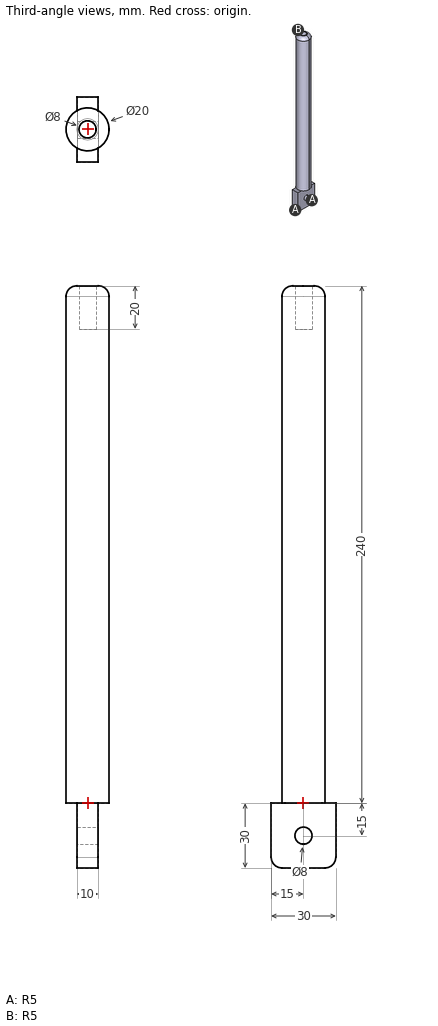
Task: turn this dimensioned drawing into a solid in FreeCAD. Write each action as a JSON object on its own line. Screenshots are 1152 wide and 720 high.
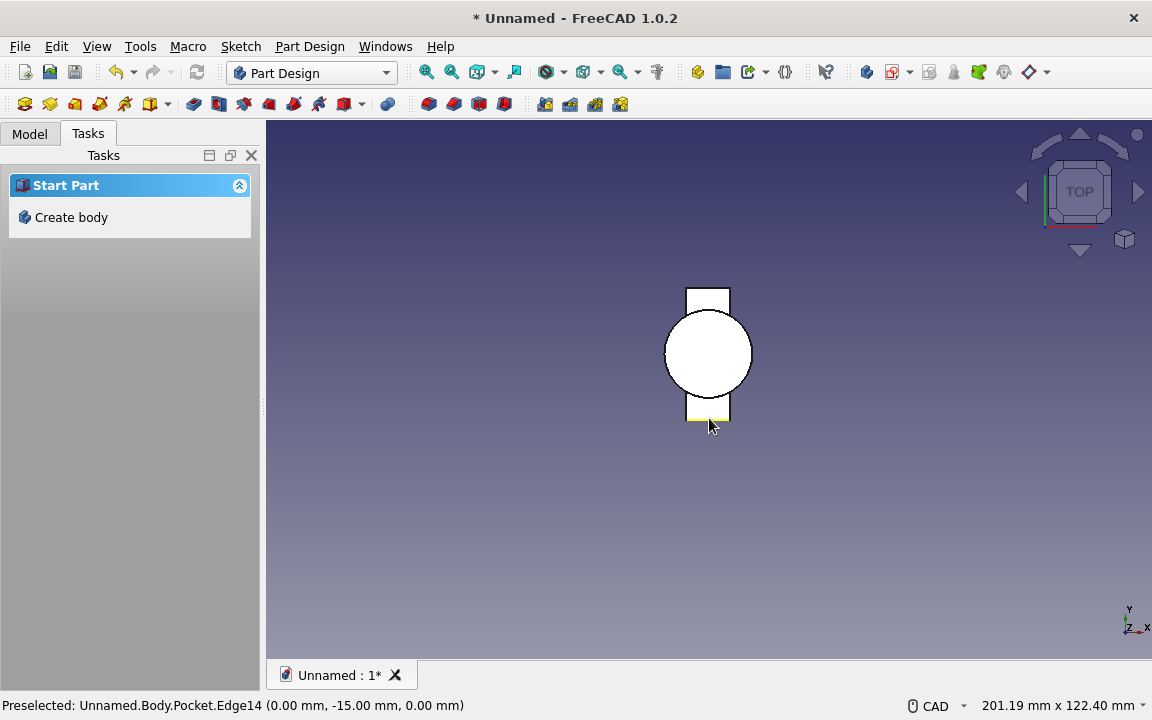
{"action": "key", "text": "v f"}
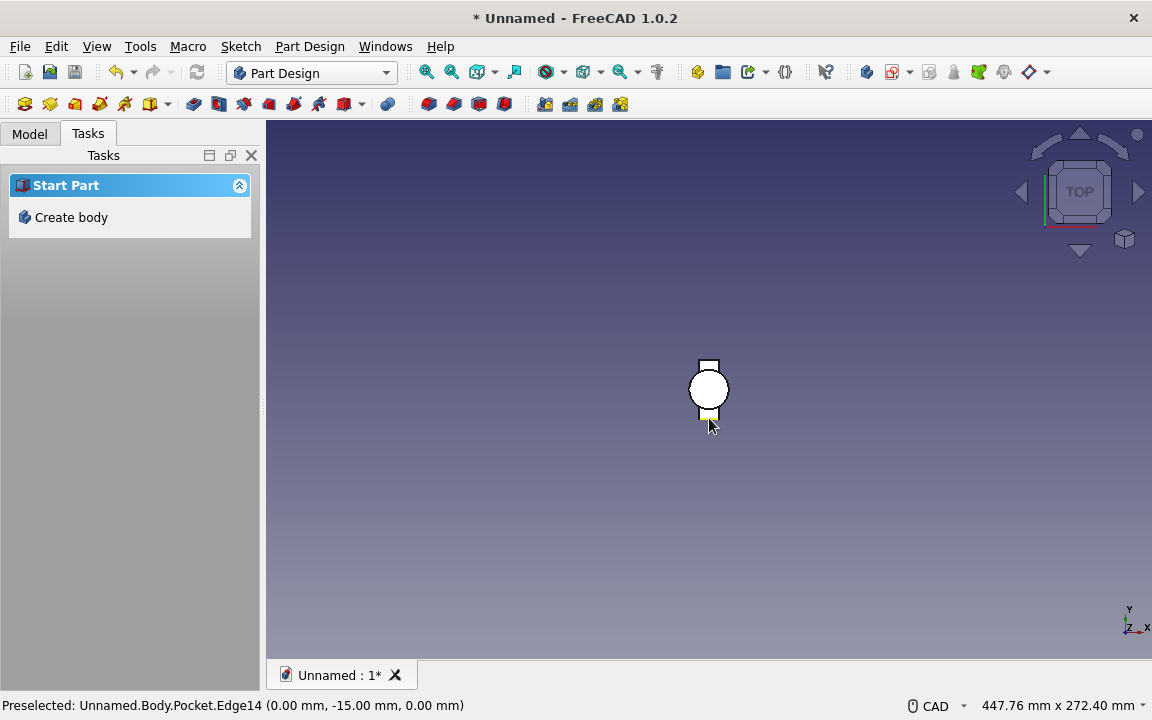
{"action": "key", "text": "1"}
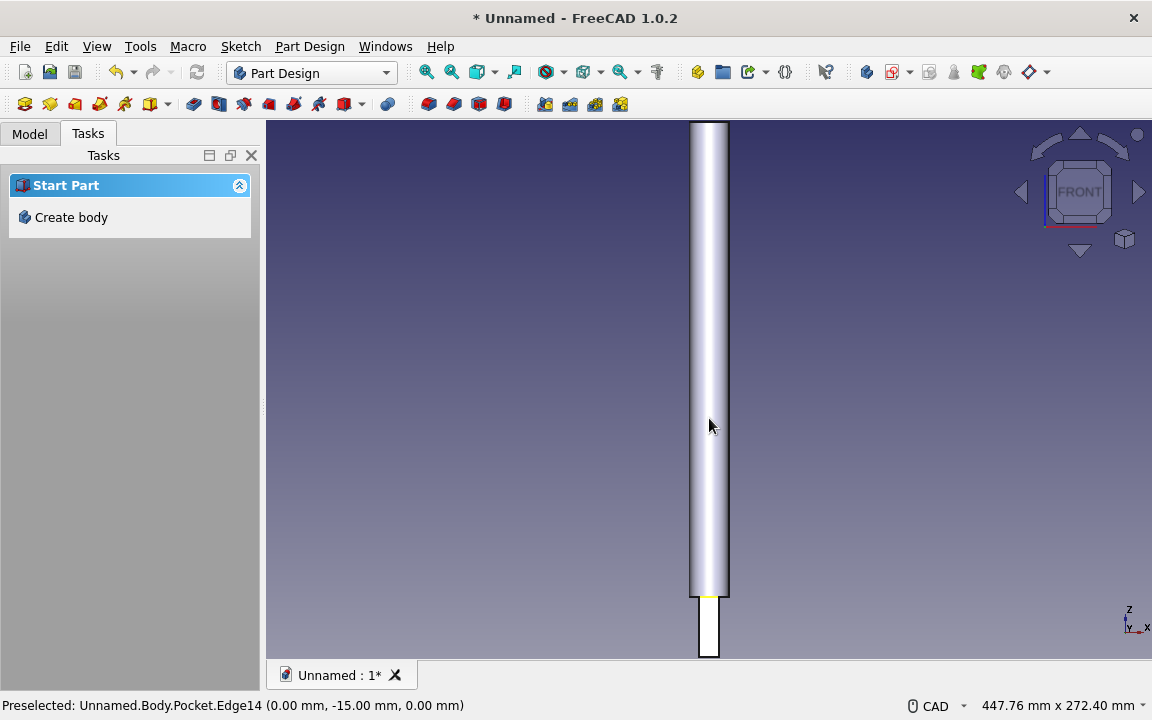
{"action": "key", "text": "3"}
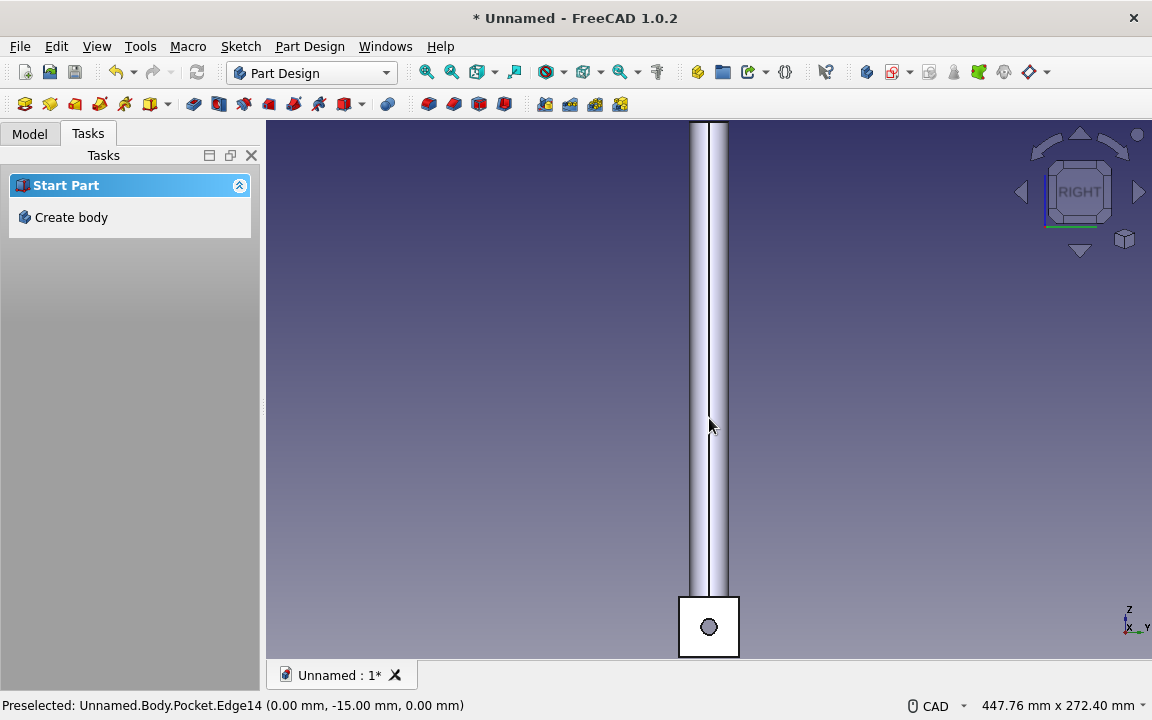
{"action": "key", "text": "5"}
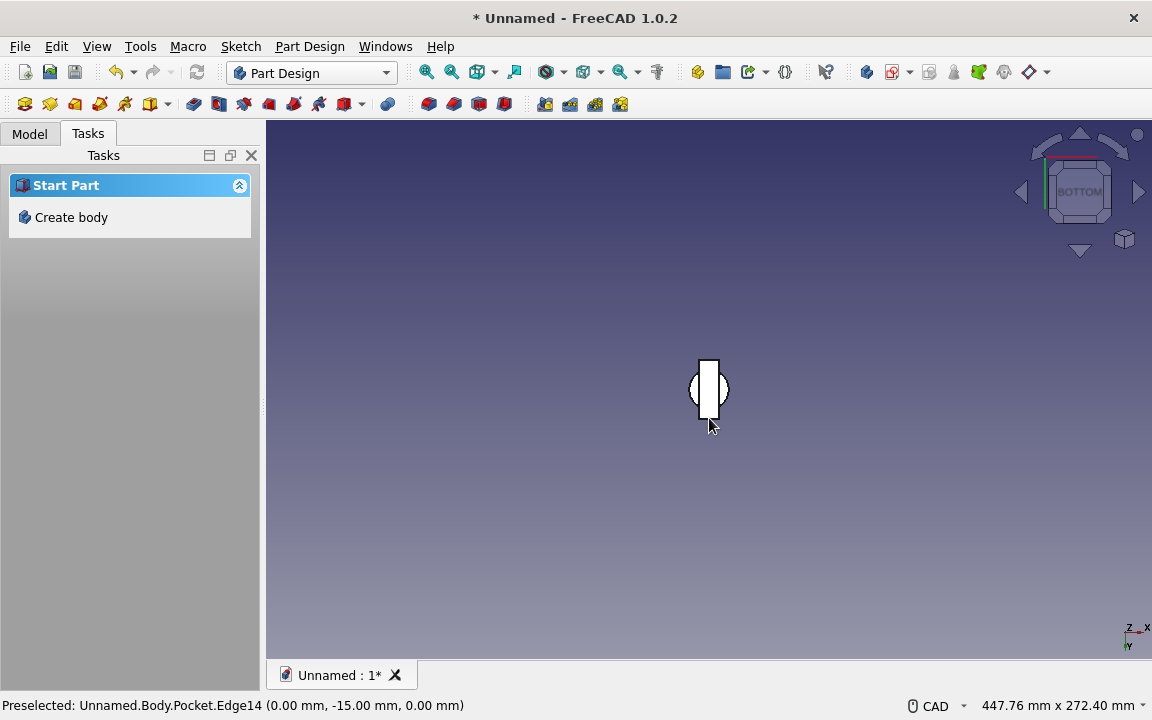
{"action": "key", "text": "v f"}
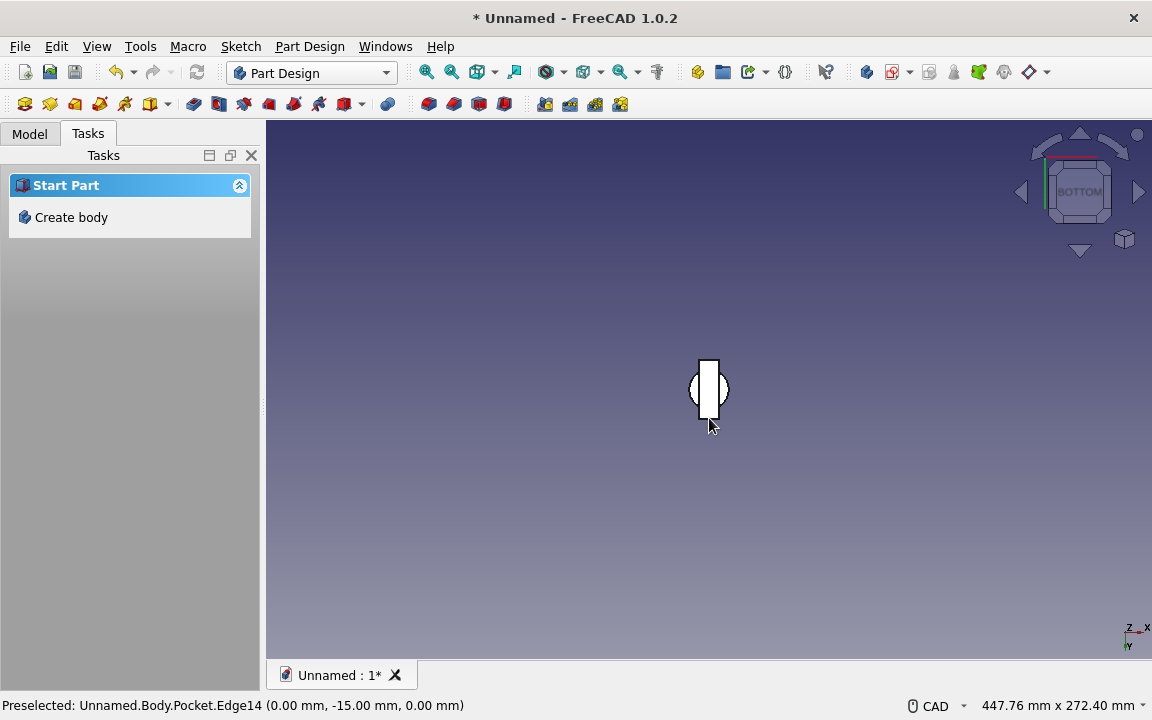
{"action": "left_click", "coordinate": [709, 359]}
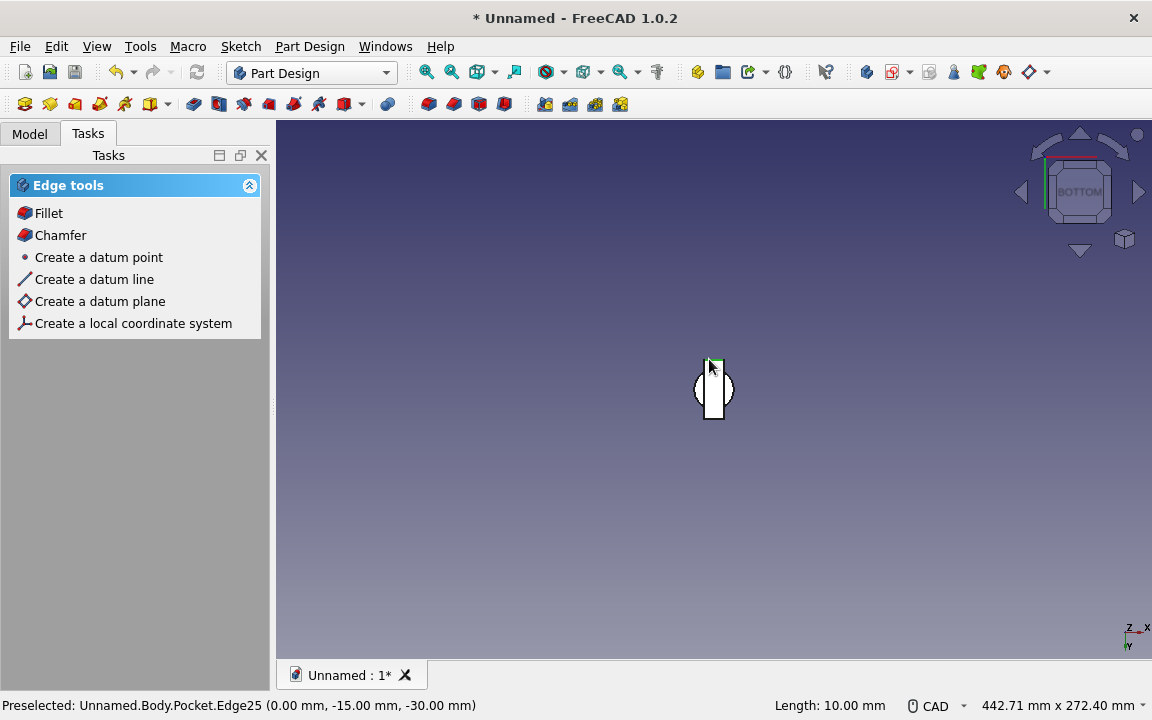
{"action": "left_click", "coordinate": [714, 418], "text": "ctrl"}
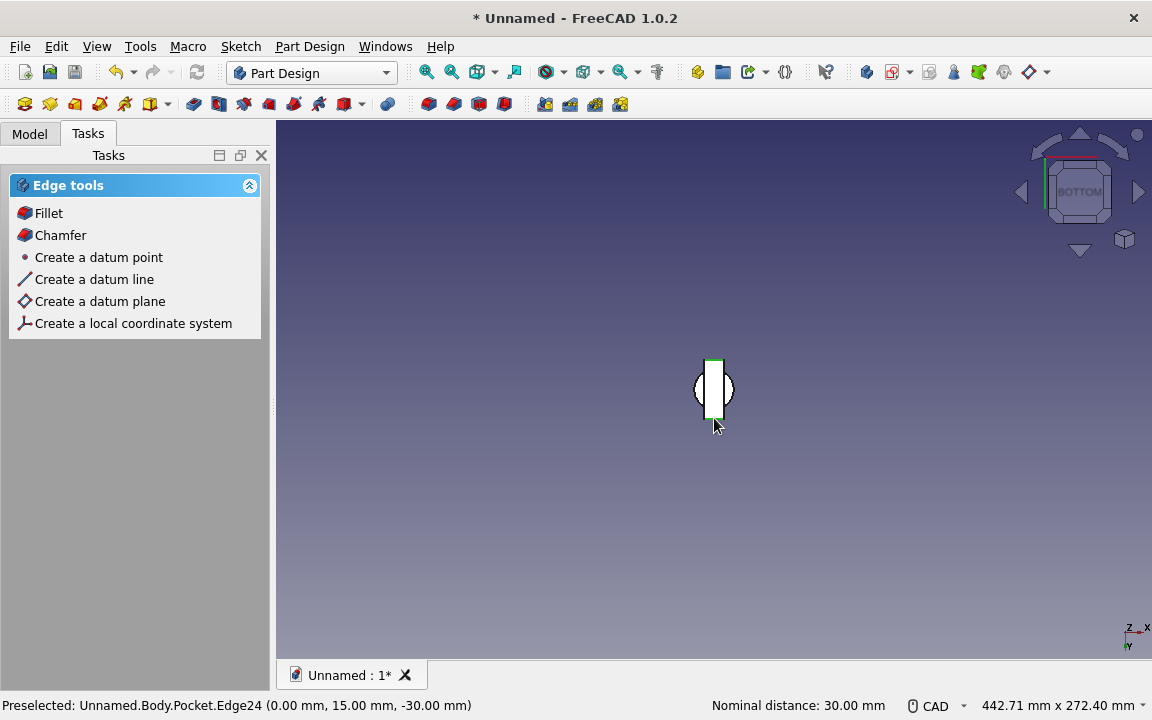
{"action": "left_click", "coordinate": [429, 104]}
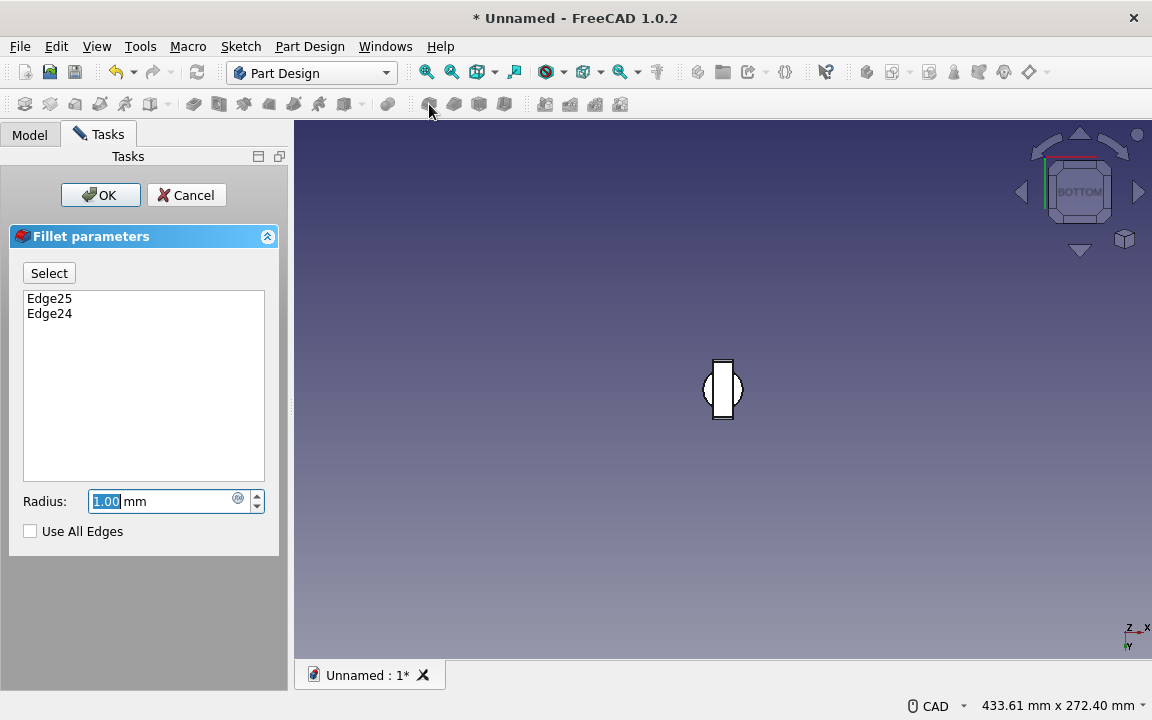
{"action": "type", "text": "5"}
{"action": "key", "text": "Tab"}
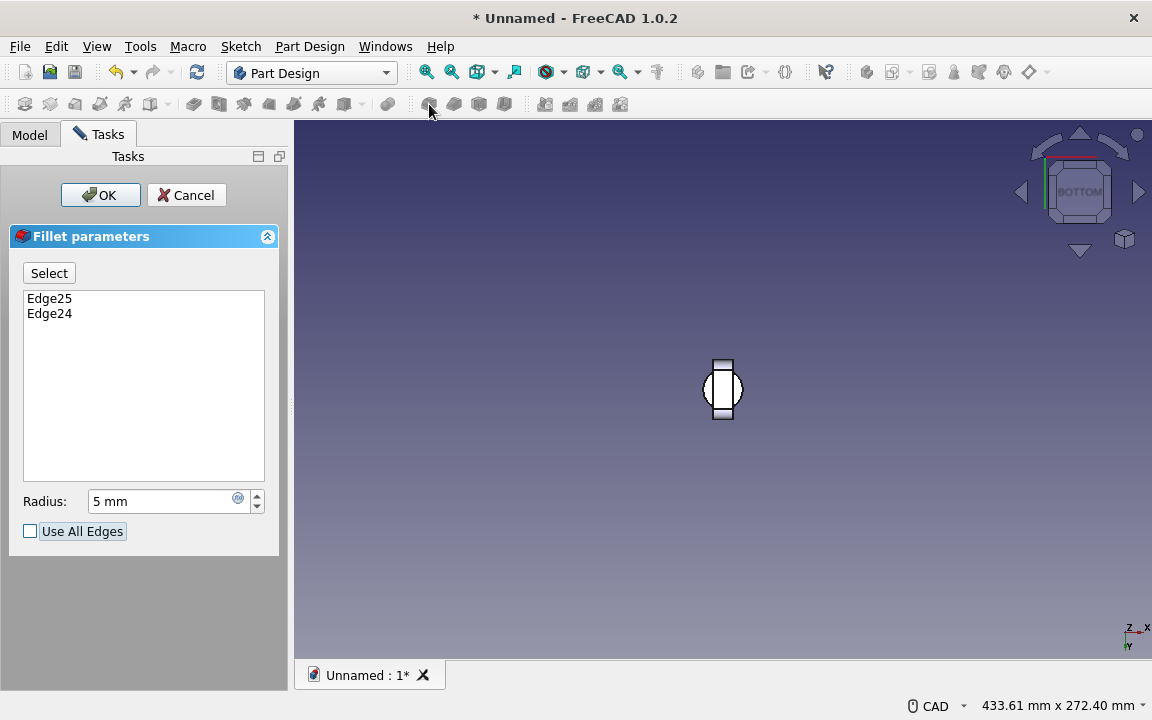
{"action": "left_click", "coordinate": [101, 195]}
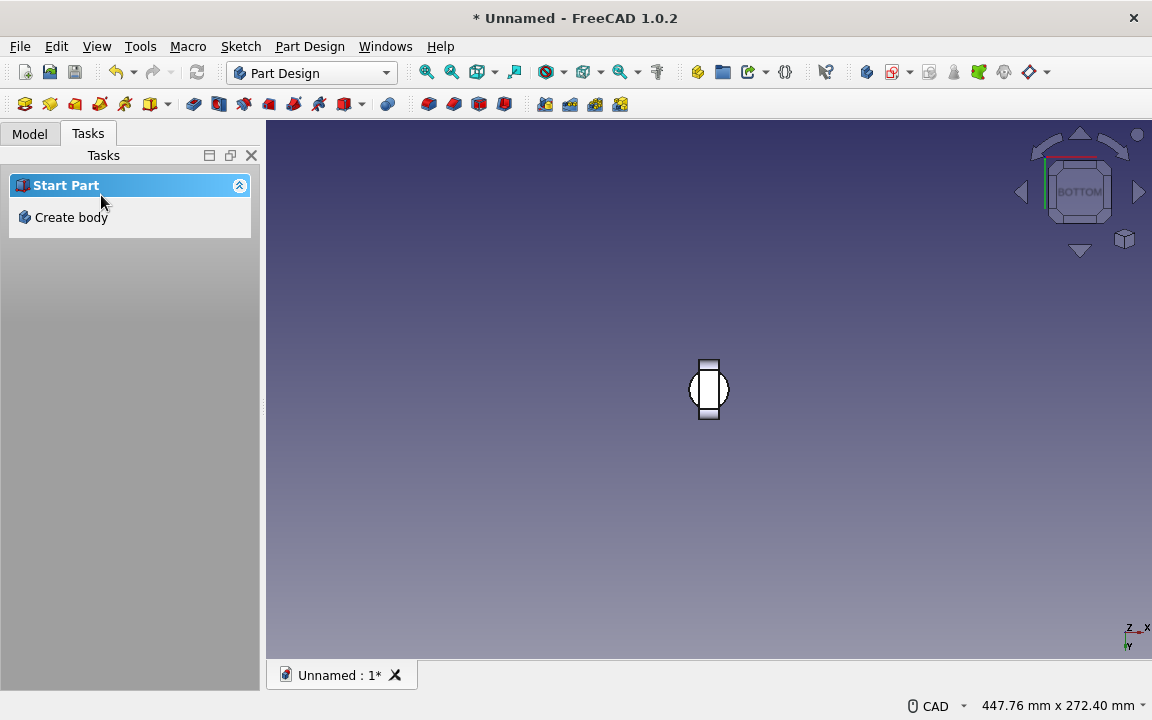
{"action": "key", "text": "v f"}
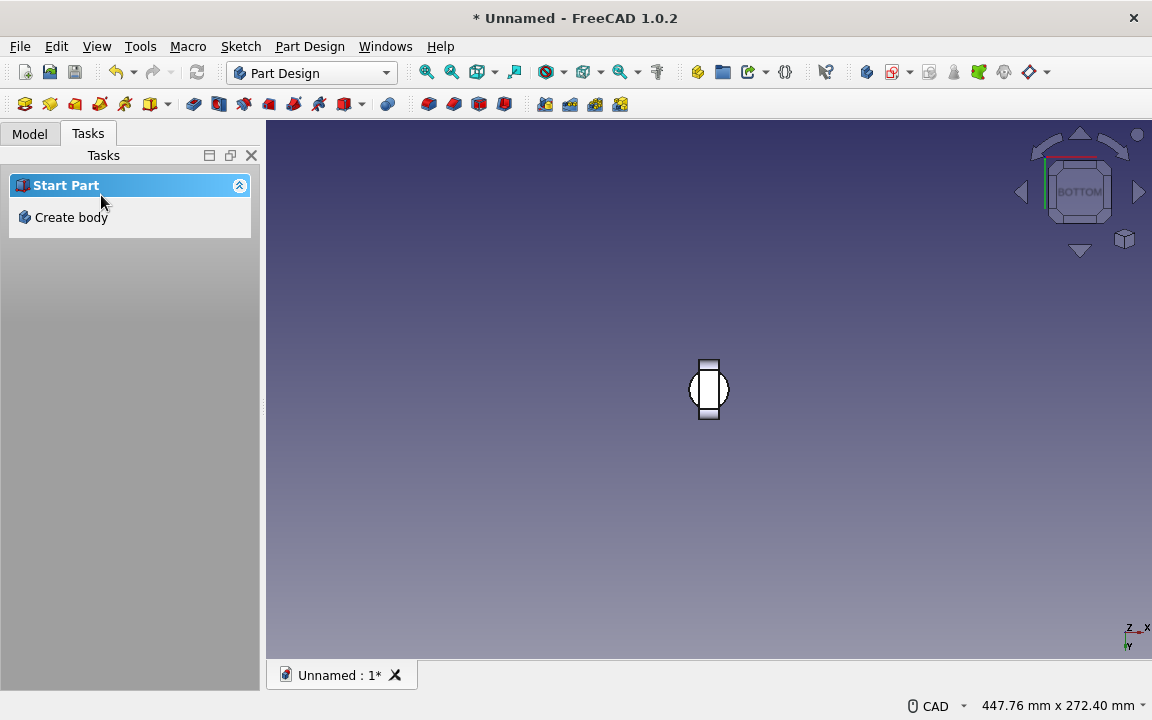
{"action": "key", "text": "0"}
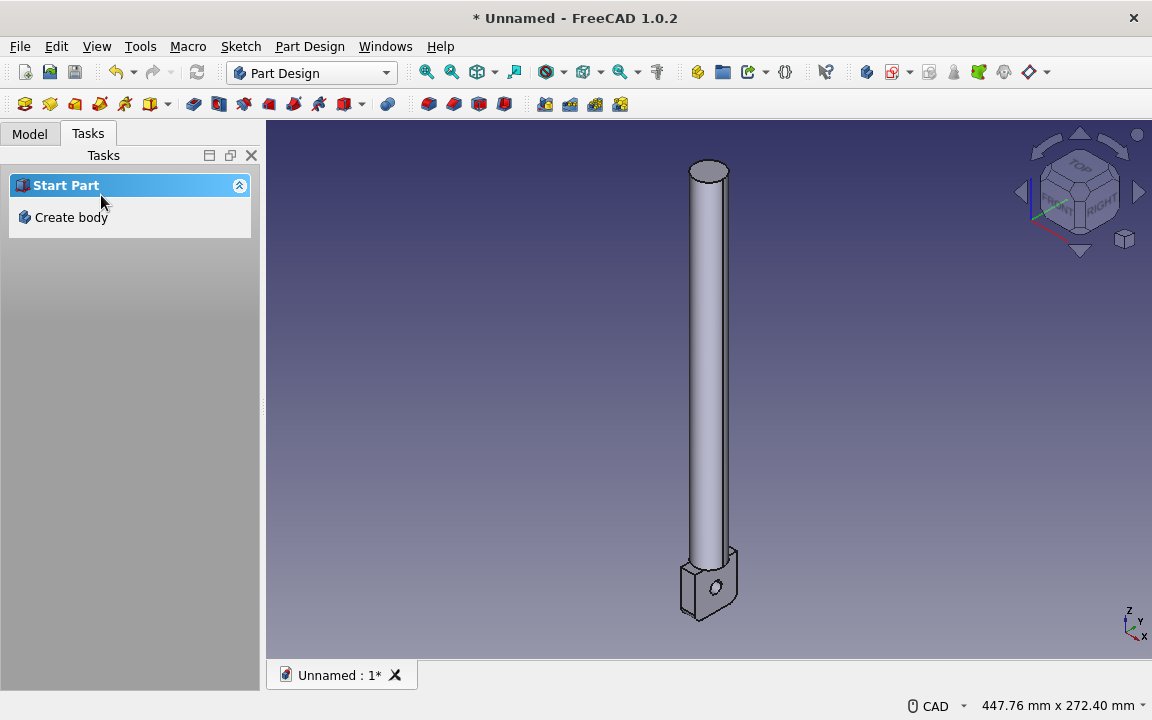
{"action": "left_click", "coordinate": [689, 169]}